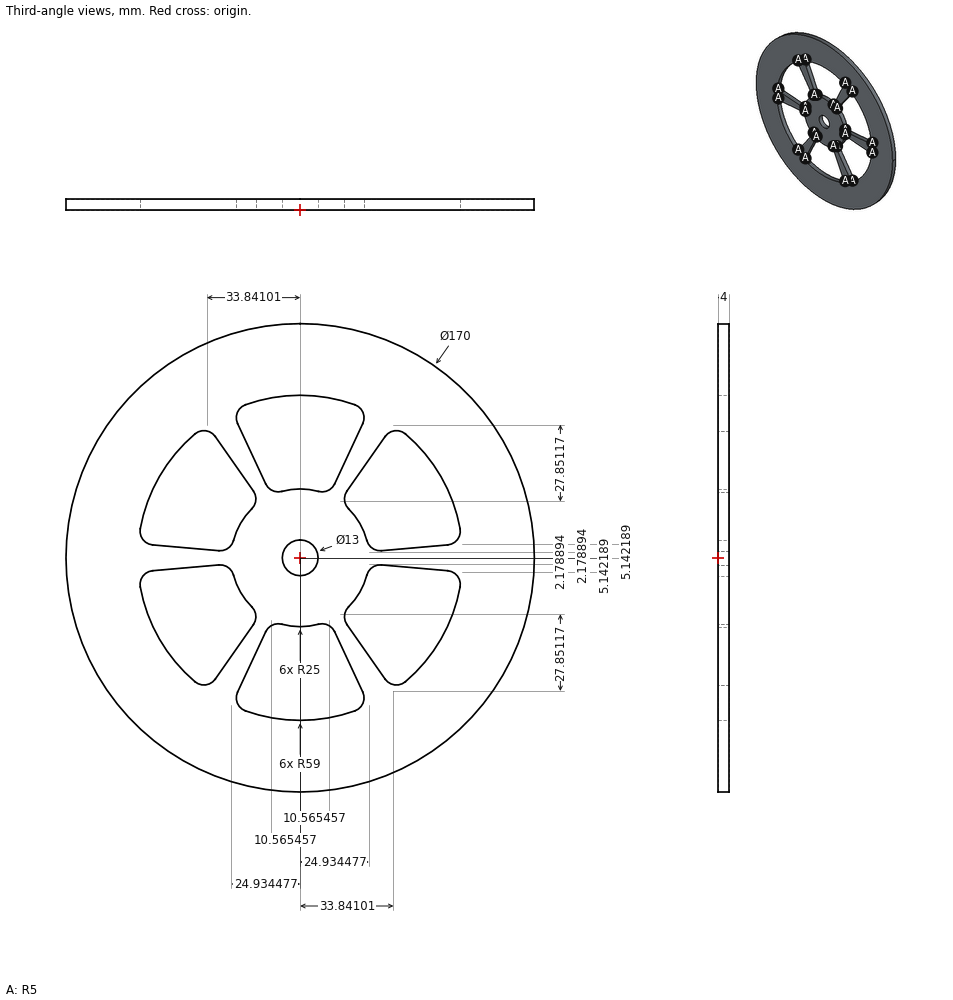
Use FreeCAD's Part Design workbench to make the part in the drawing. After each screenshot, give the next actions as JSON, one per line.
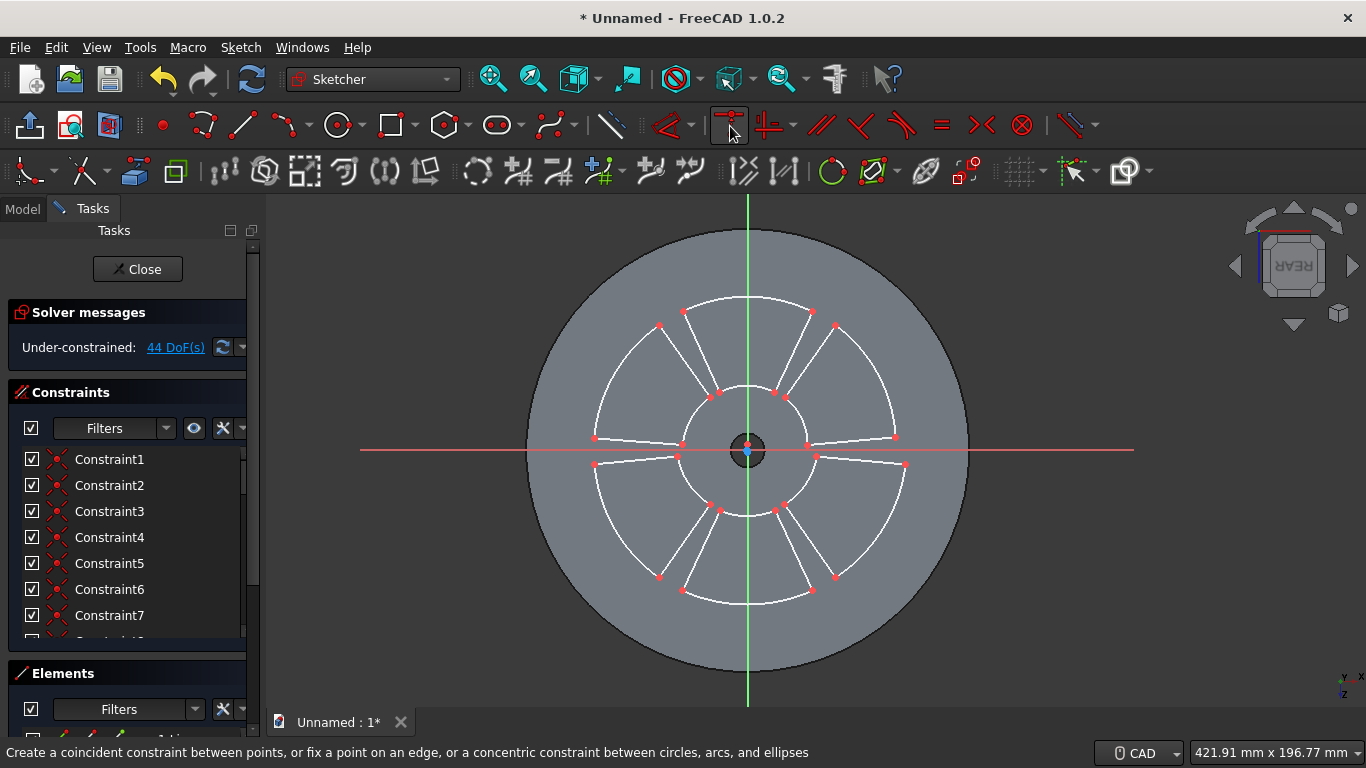
{"action": "left_click", "coordinate": [775, 299]}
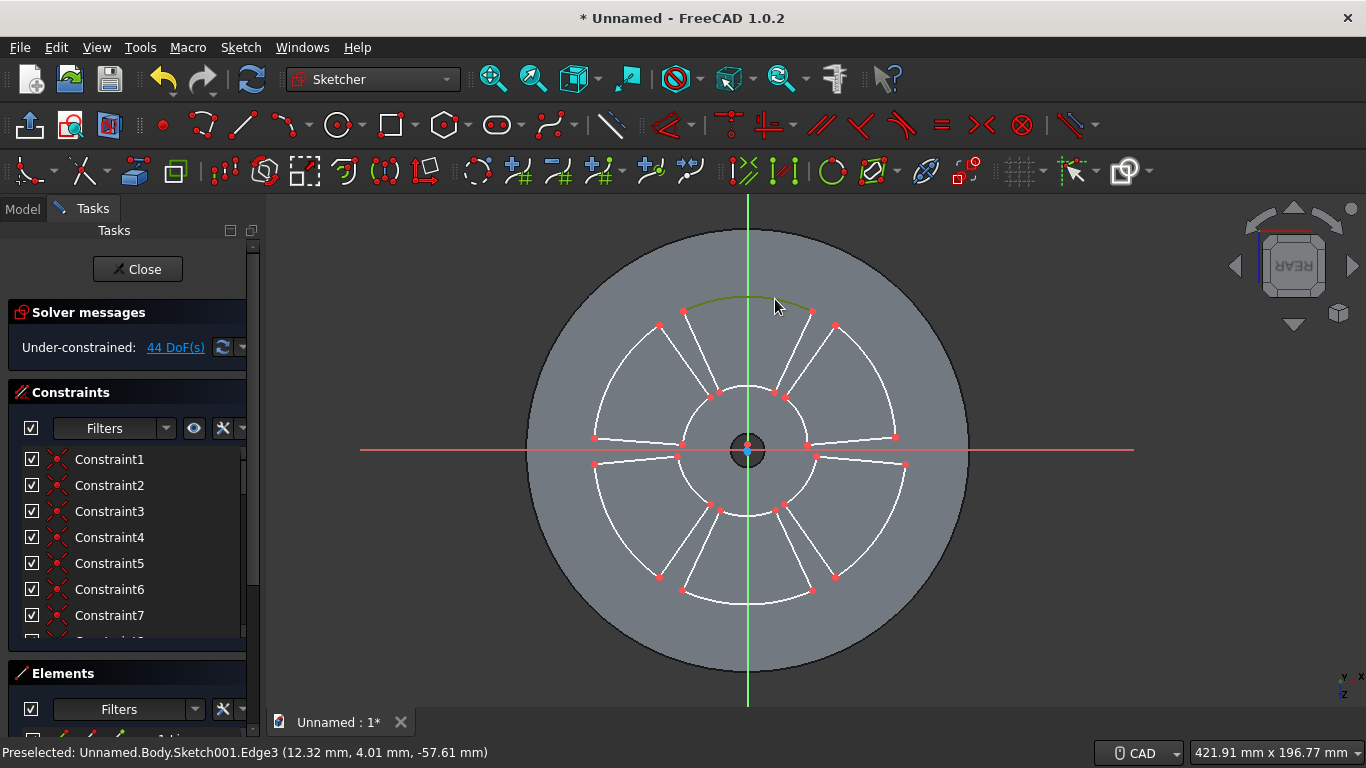
{"action": "left_click", "coordinate": [603, 504]}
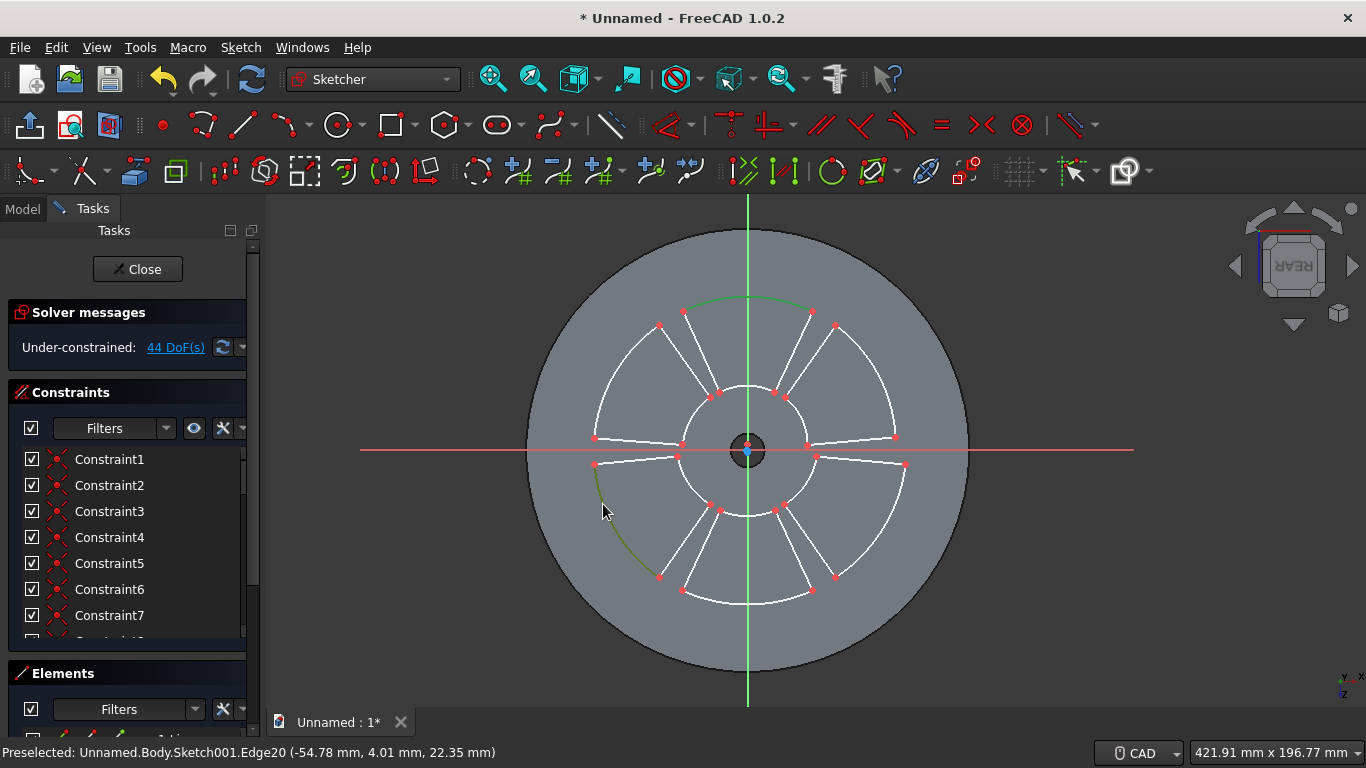
{"action": "left_click", "coordinate": [730, 126]}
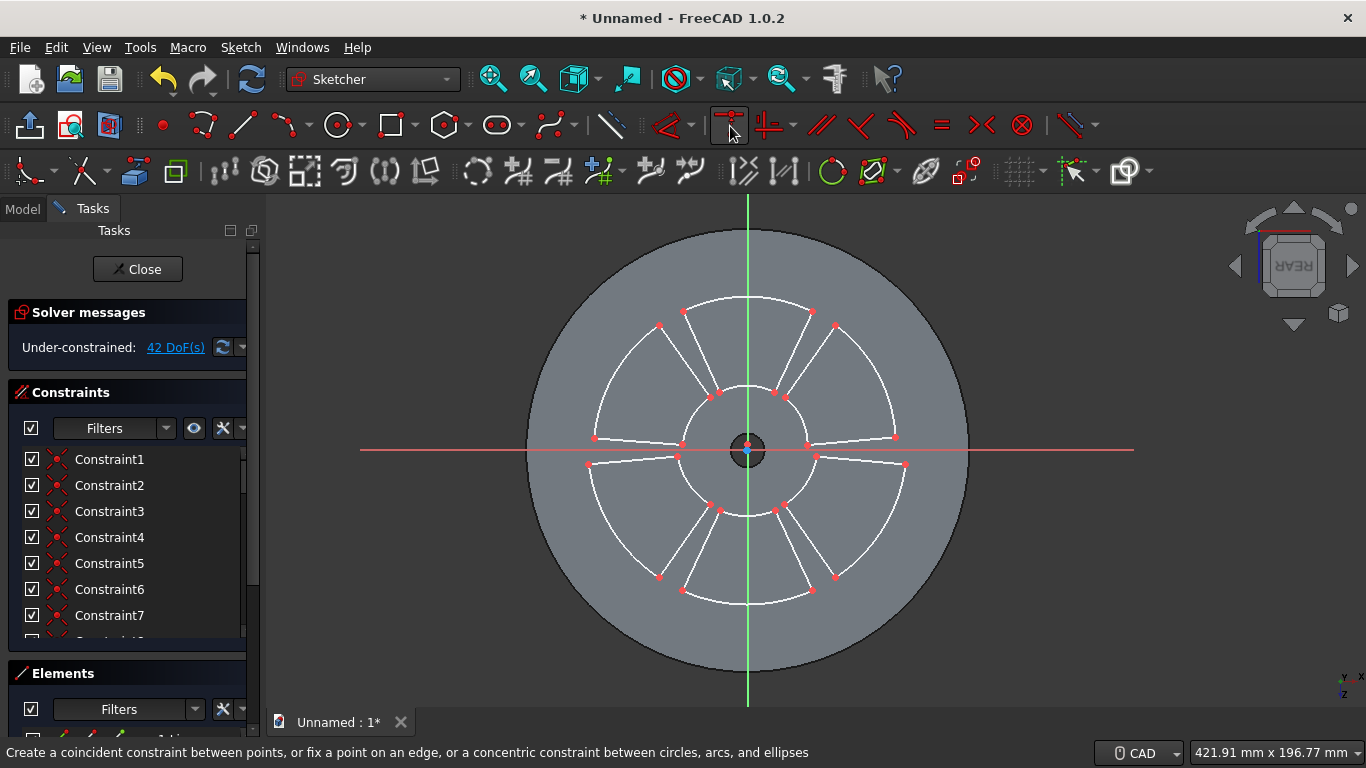
{"action": "left_click", "coordinate": [775, 299]}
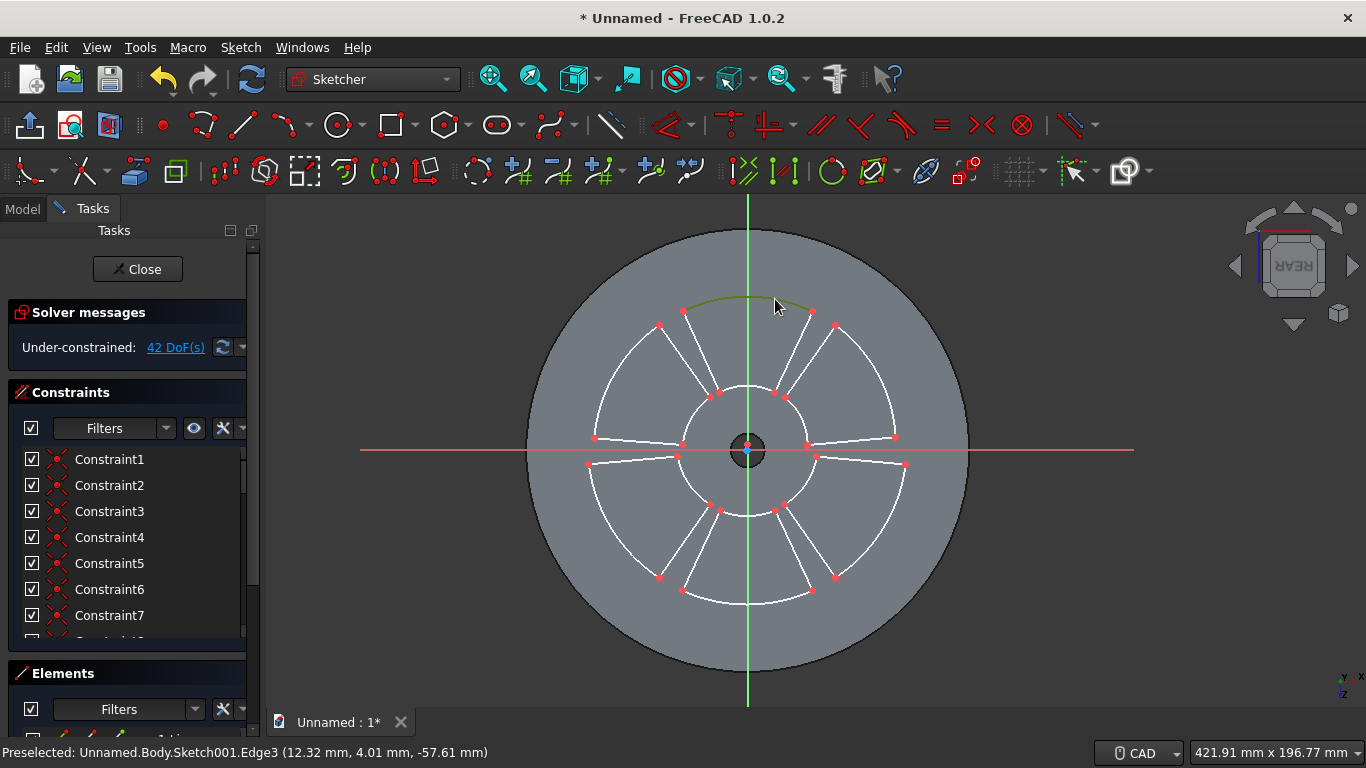
{"action": "left_click", "coordinate": [698, 409]}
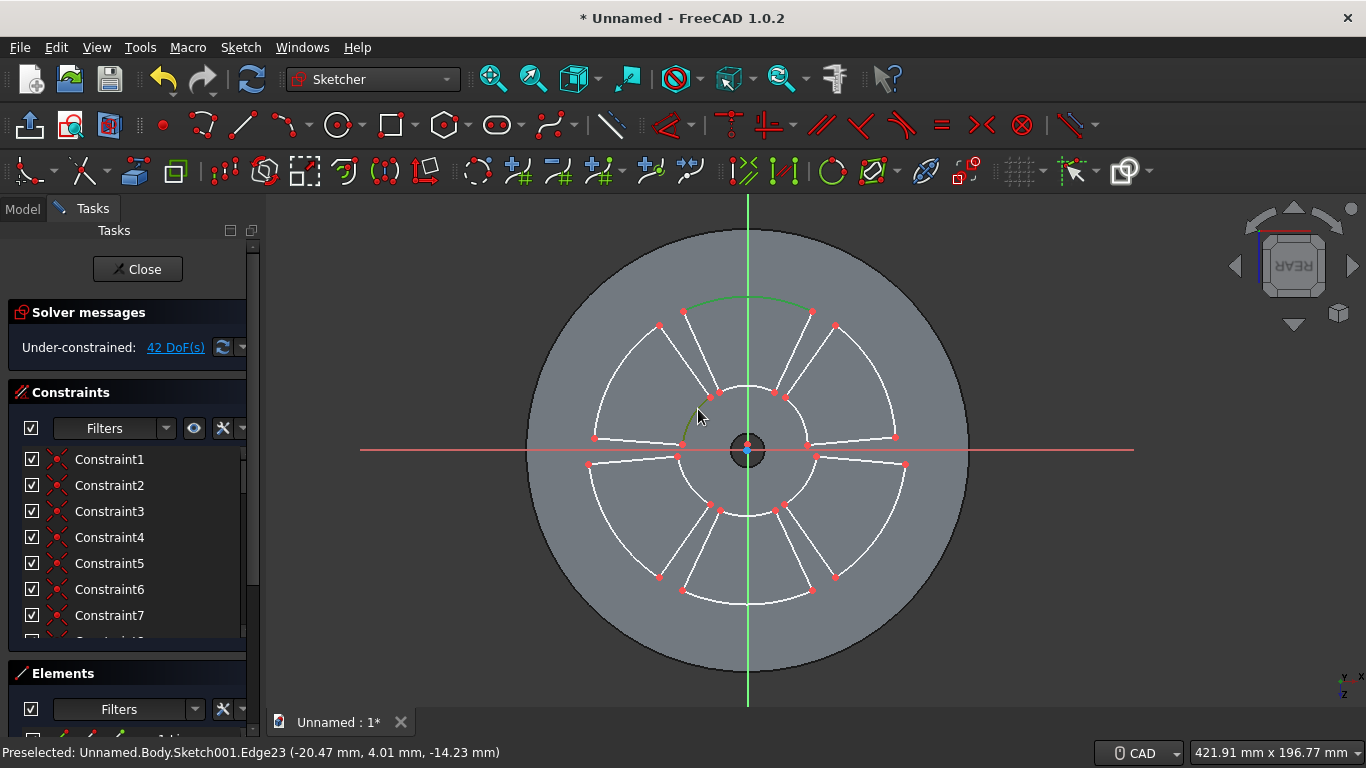
{"action": "left_click", "coordinate": [730, 126]}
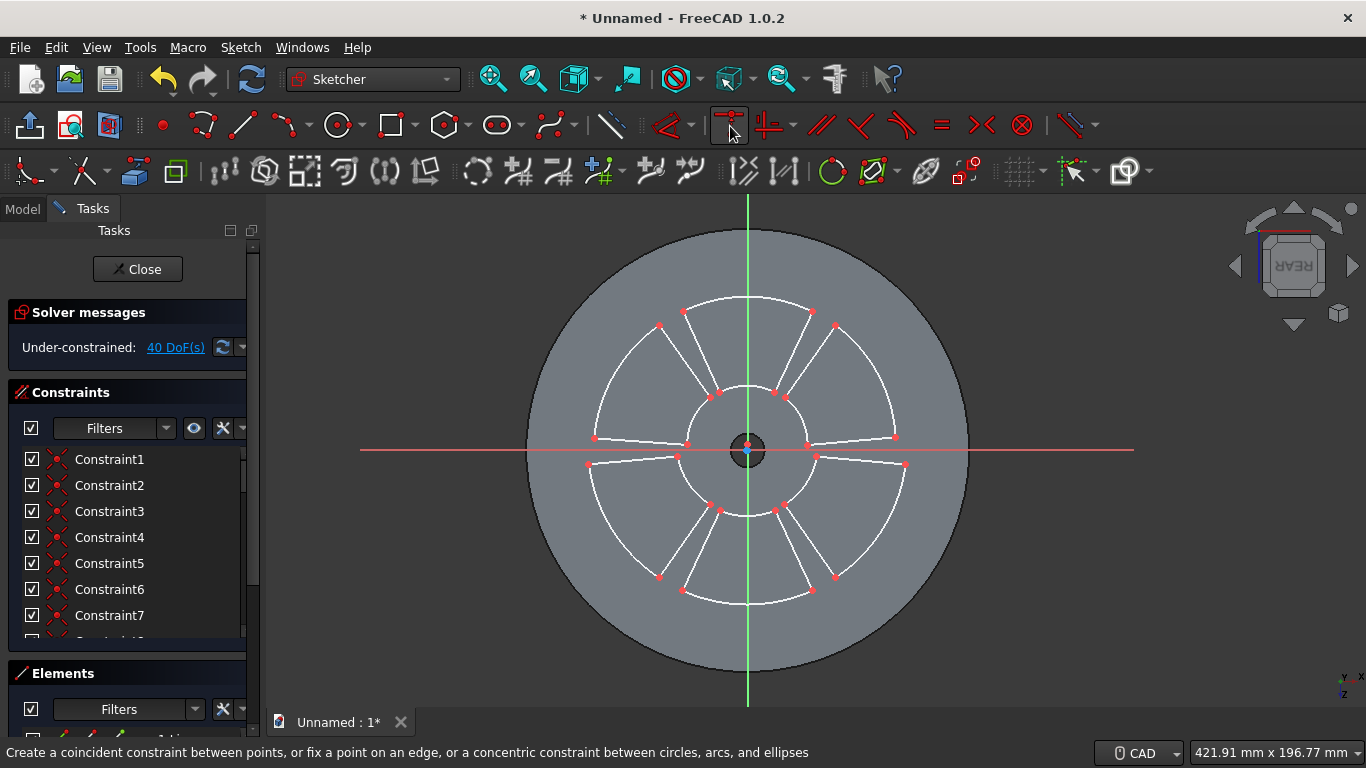
{"action": "left_click", "coordinate": [775, 299]}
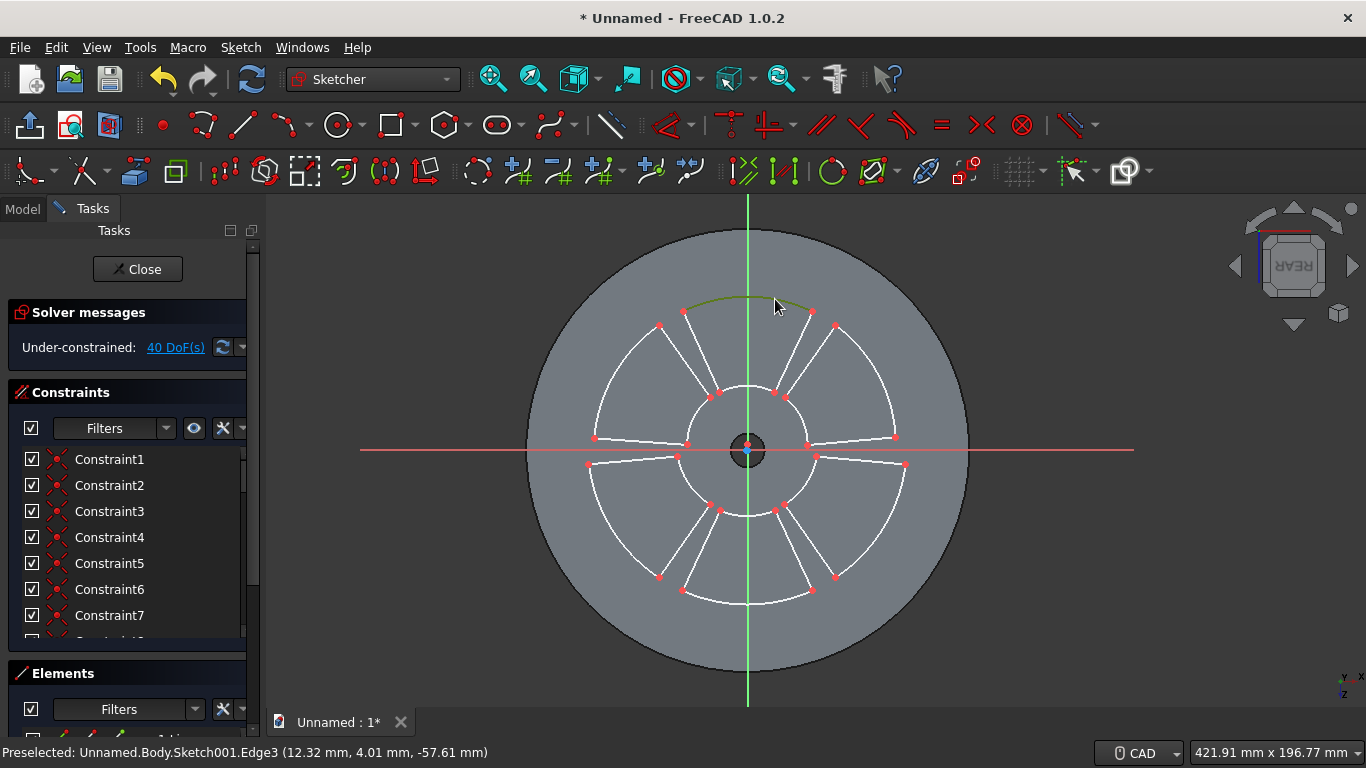
{"action": "left_click", "coordinate": [630, 353]}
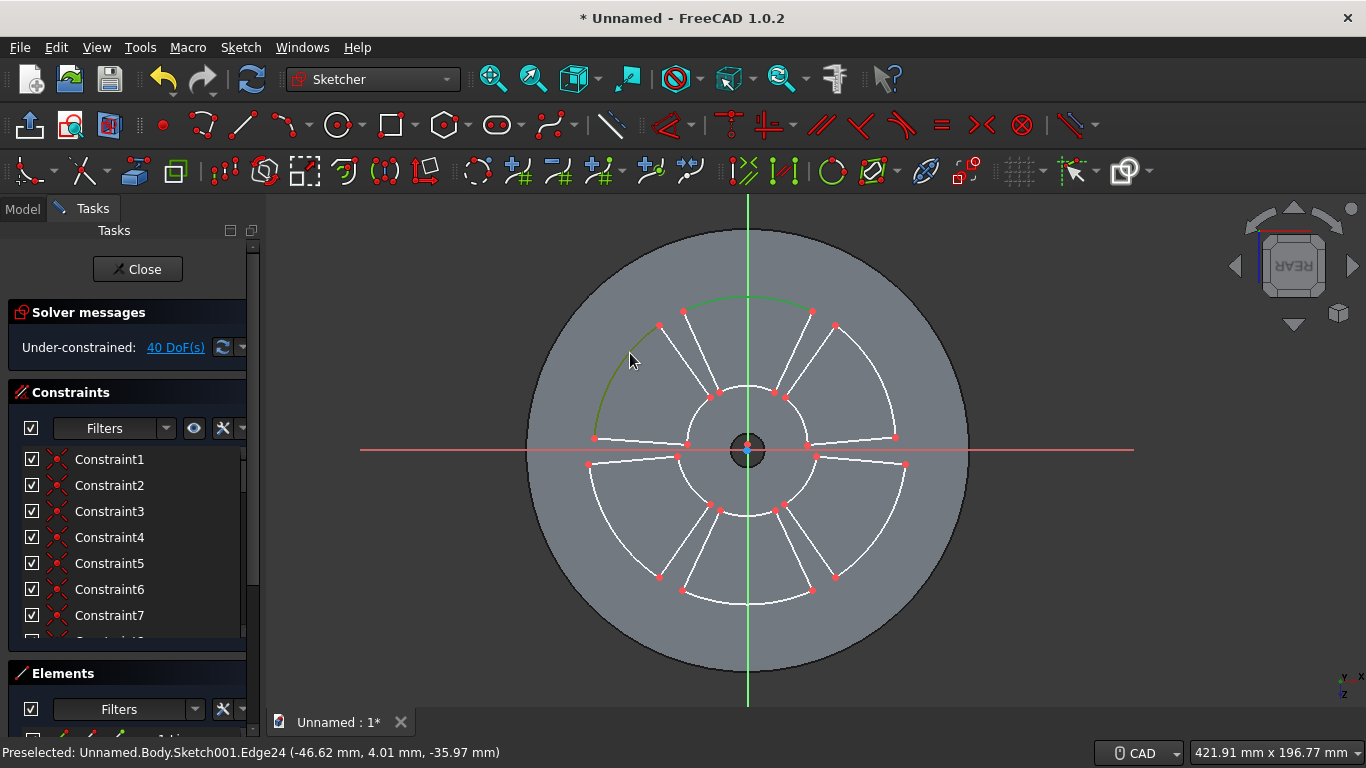
{"action": "left_click", "coordinate": [730, 126]}